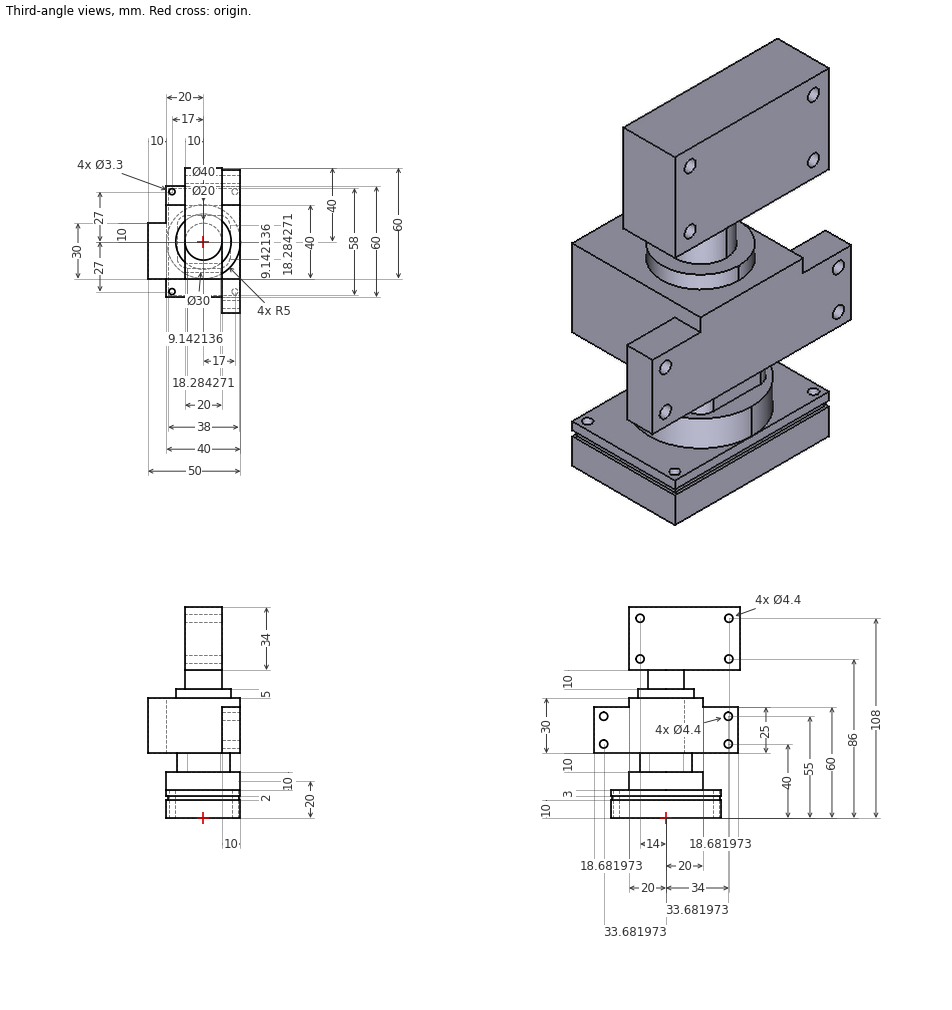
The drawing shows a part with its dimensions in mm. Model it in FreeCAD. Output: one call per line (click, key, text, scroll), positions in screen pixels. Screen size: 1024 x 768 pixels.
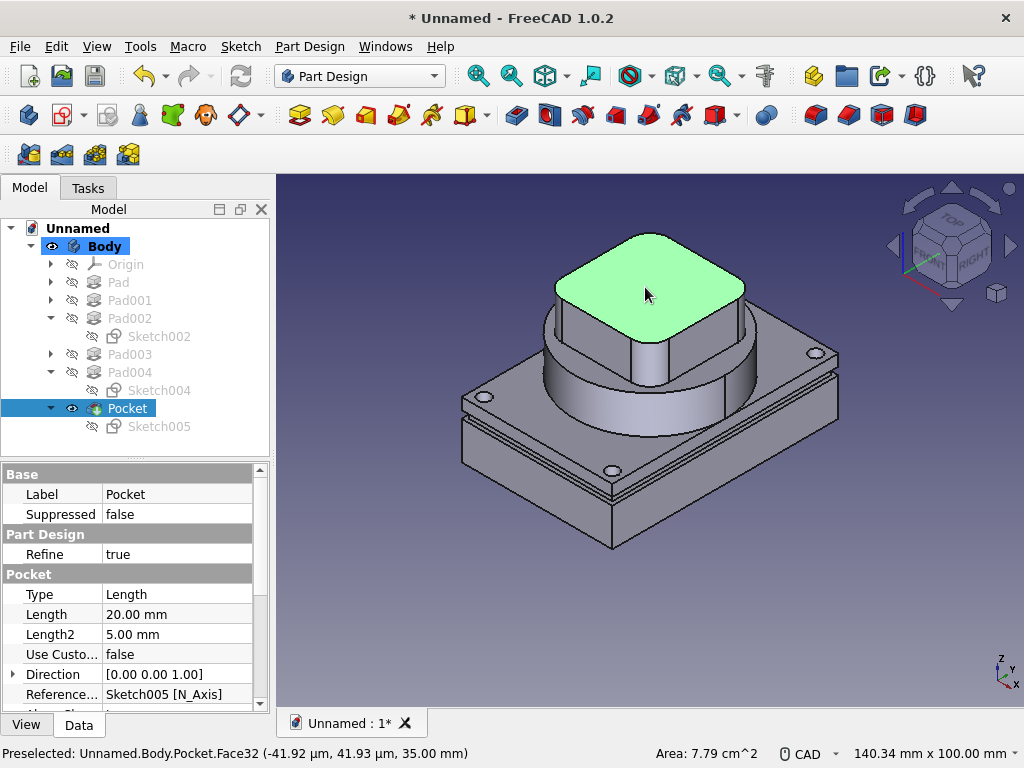
click(62, 116)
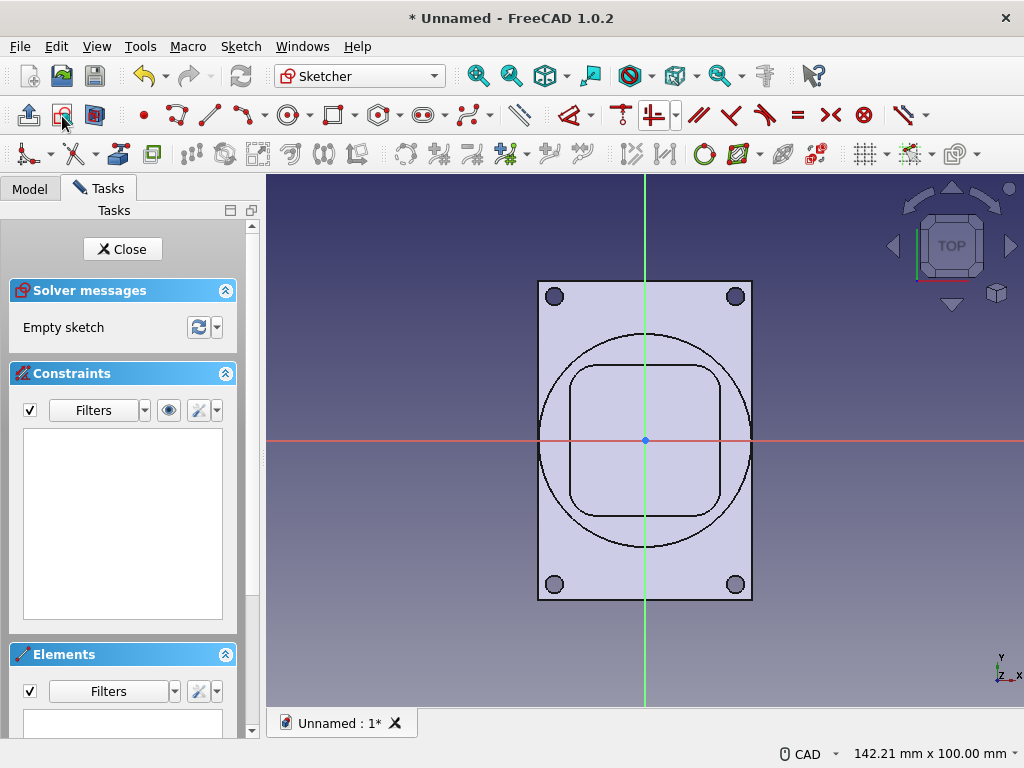
scroll(703, 440, up, 2)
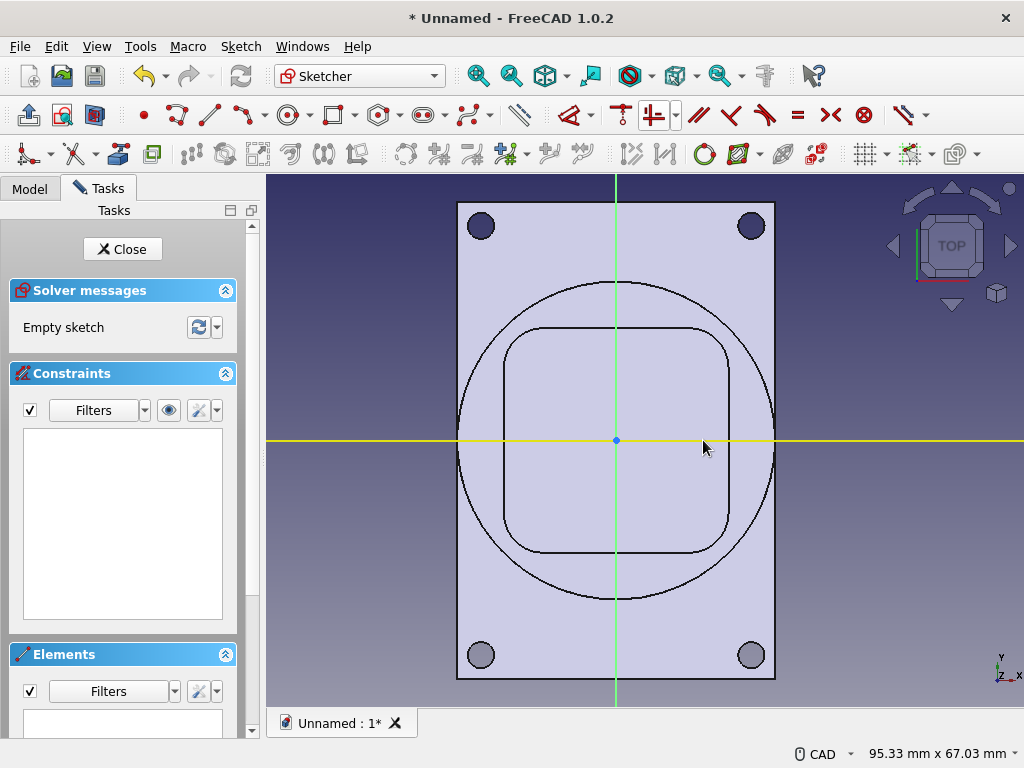
key(g)
key(m)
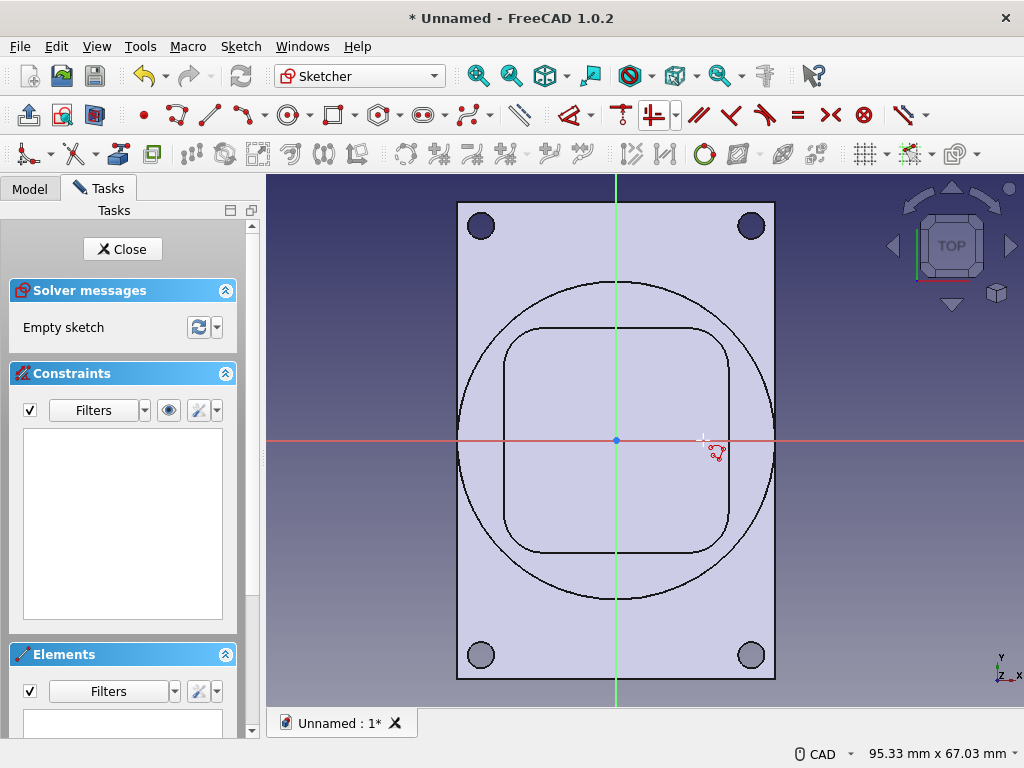
click(457, 361)
click(378, 361)
click(378, 600)
click(775, 600)
click(775, 281)
click(457, 281)
click(457, 362)
key(Escape)
key(Escape)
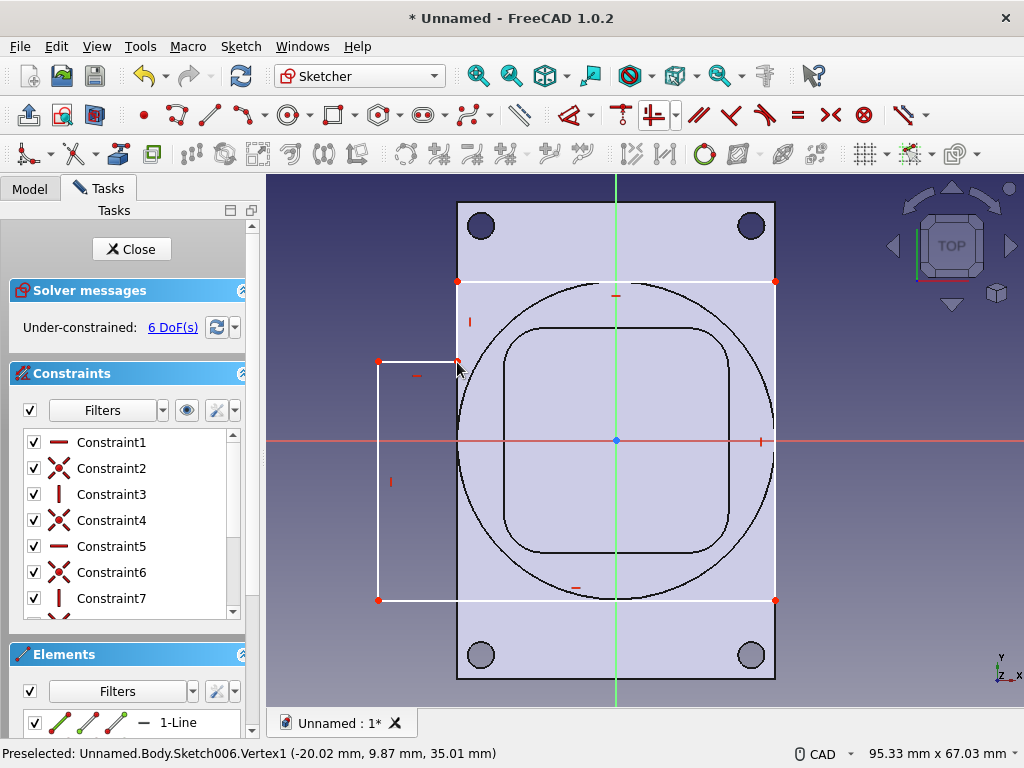
key(d)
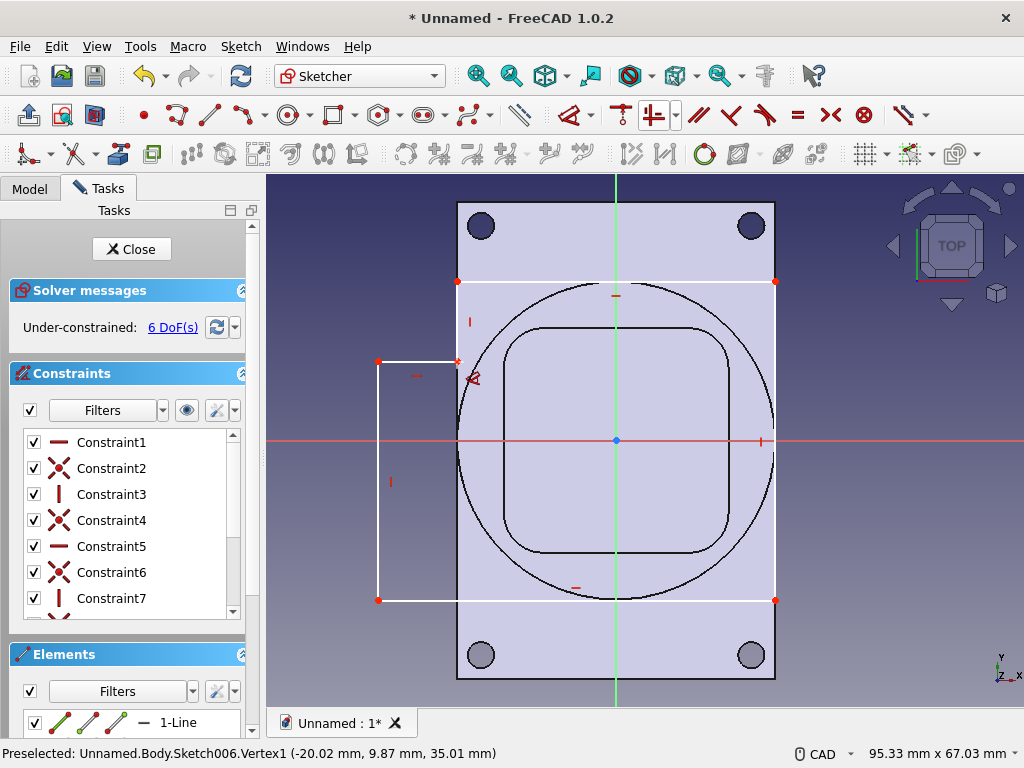
click(433, 362)
click(418, 328)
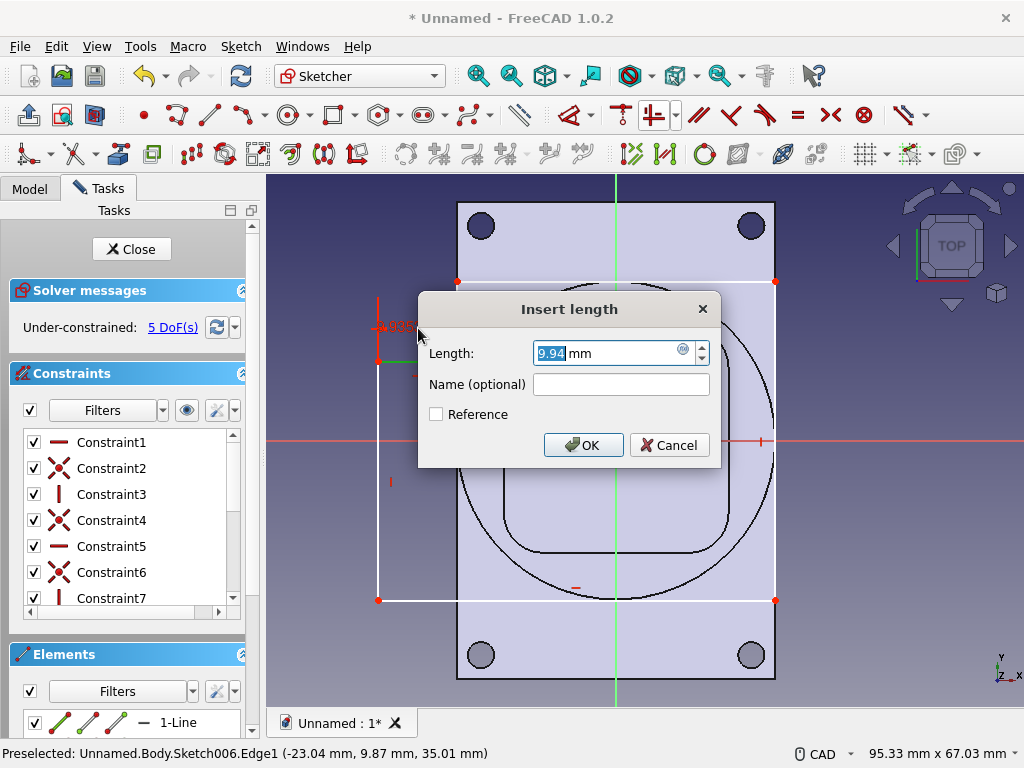
text(10)
key(Return)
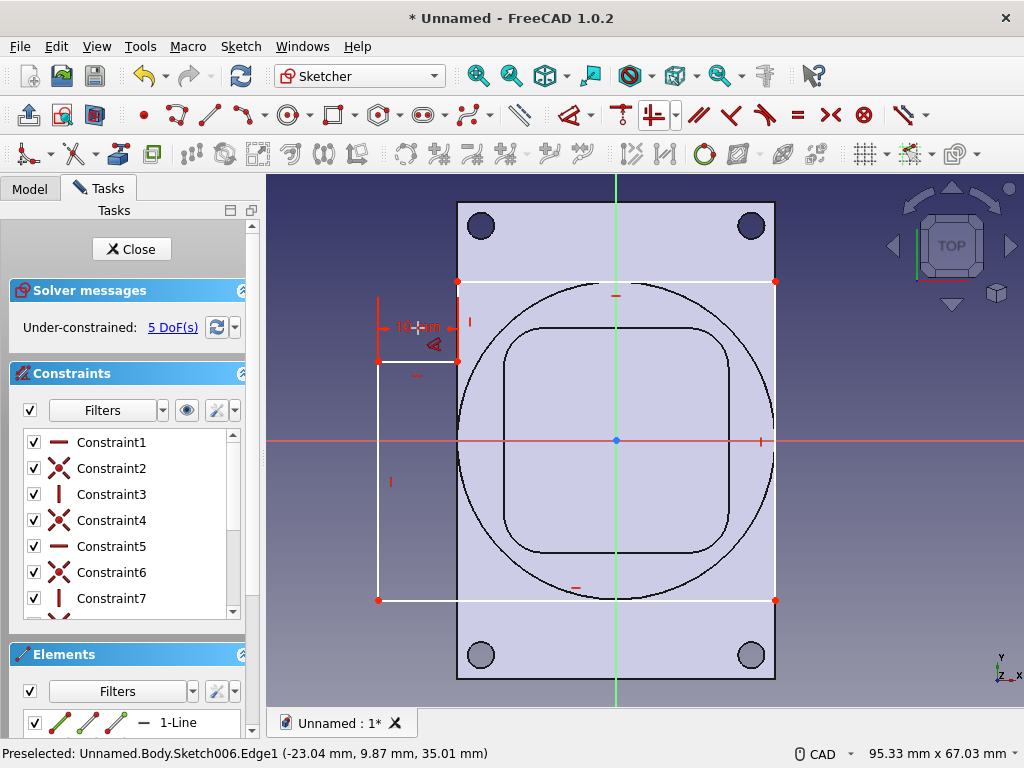
click(378, 529)
click(344, 481)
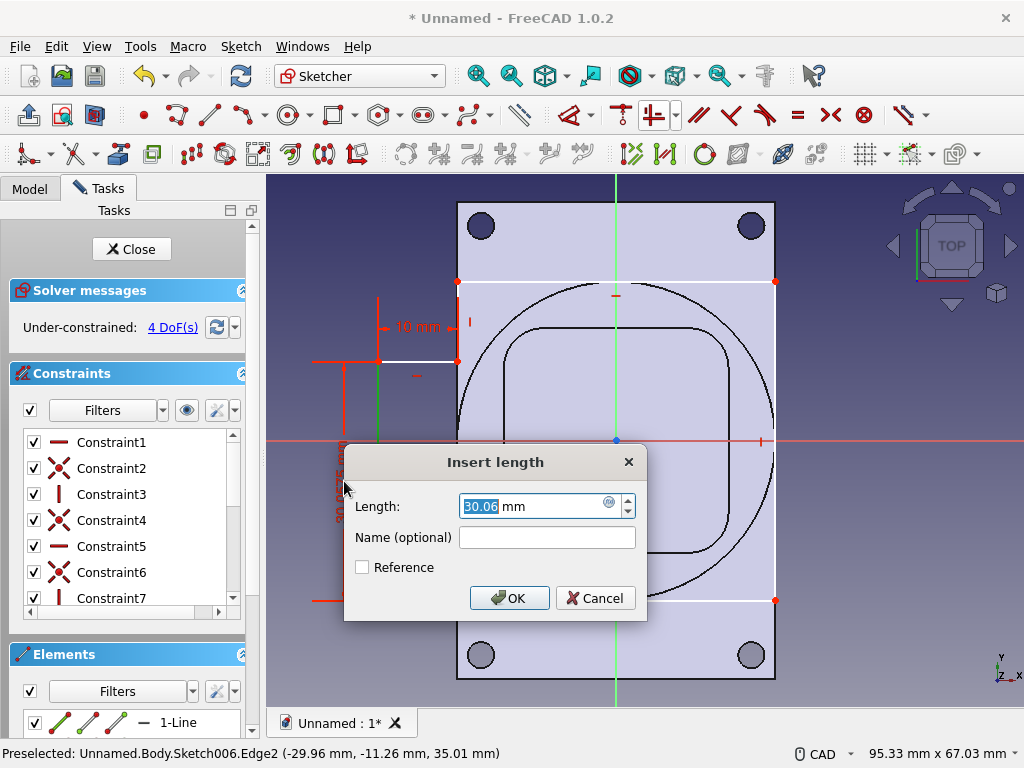
text(30)
key(Return)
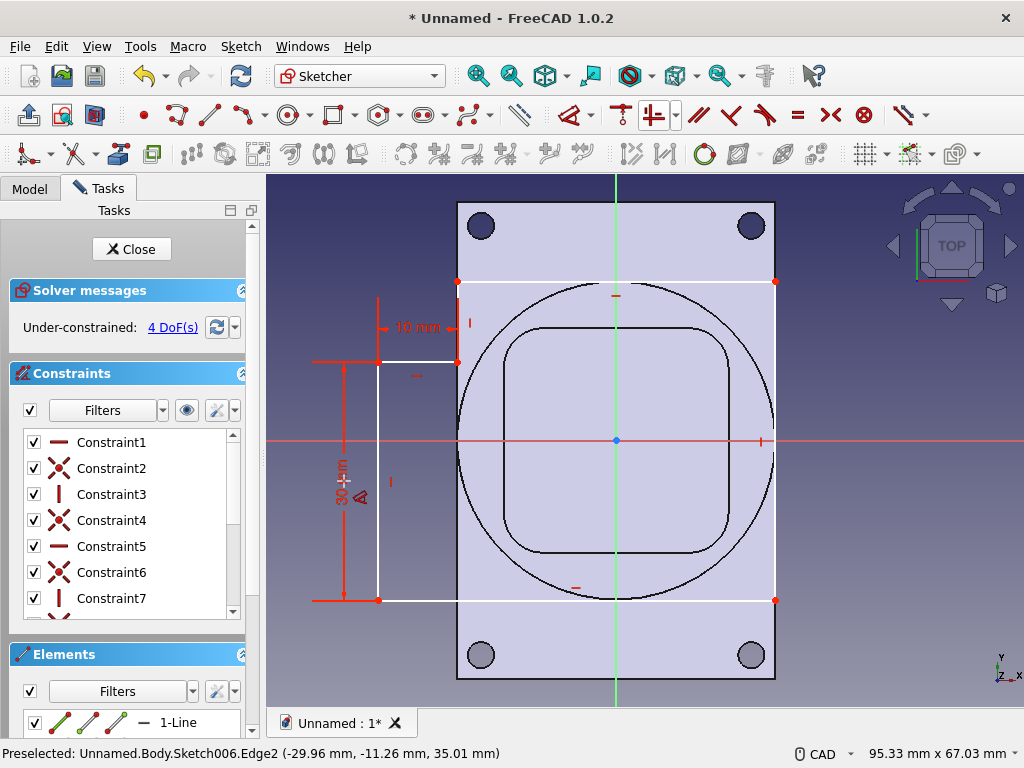
click(497, 601)
click(577, 635)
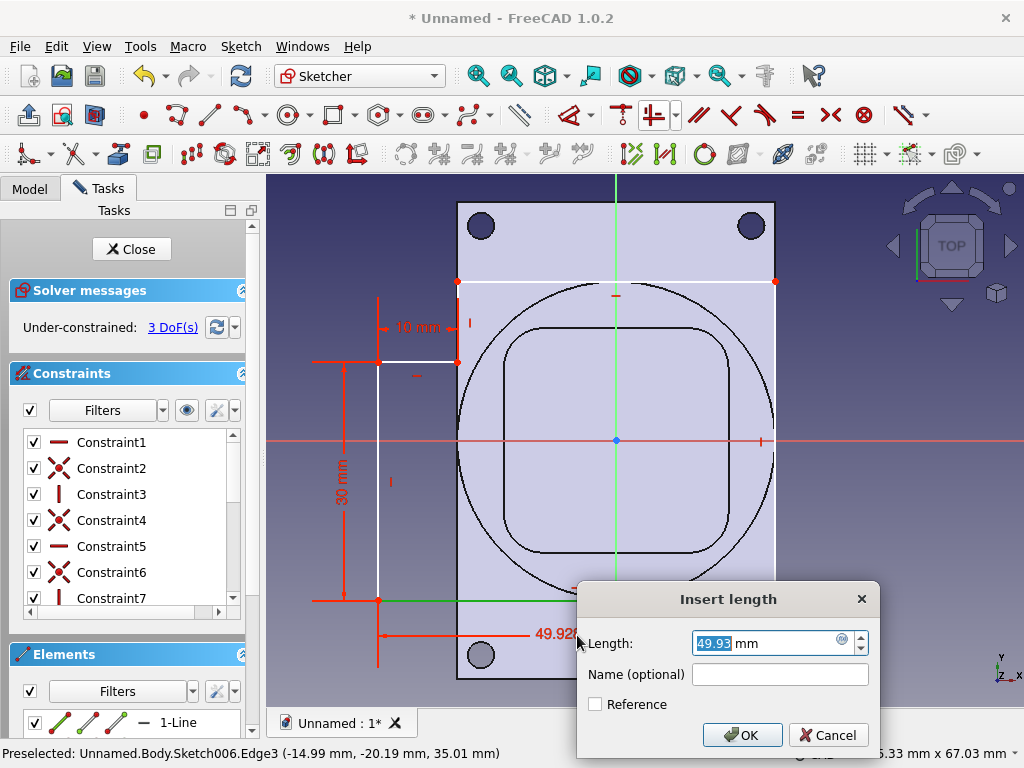
text(50)
key(Return)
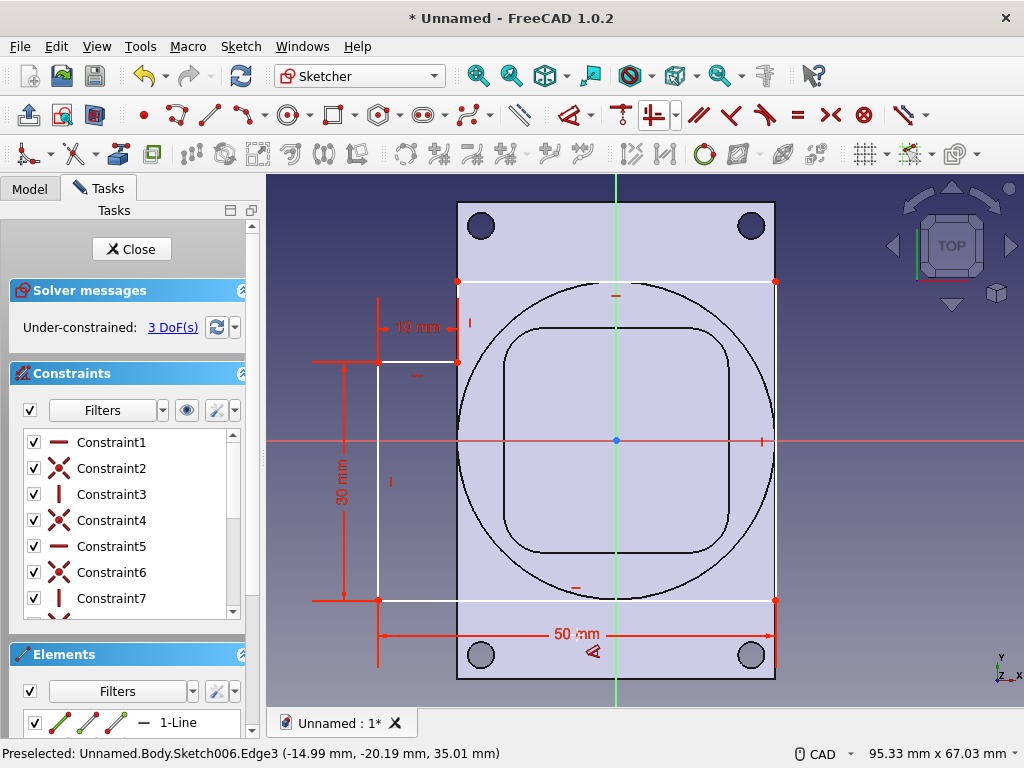
click(776, 505)
click(810, 368)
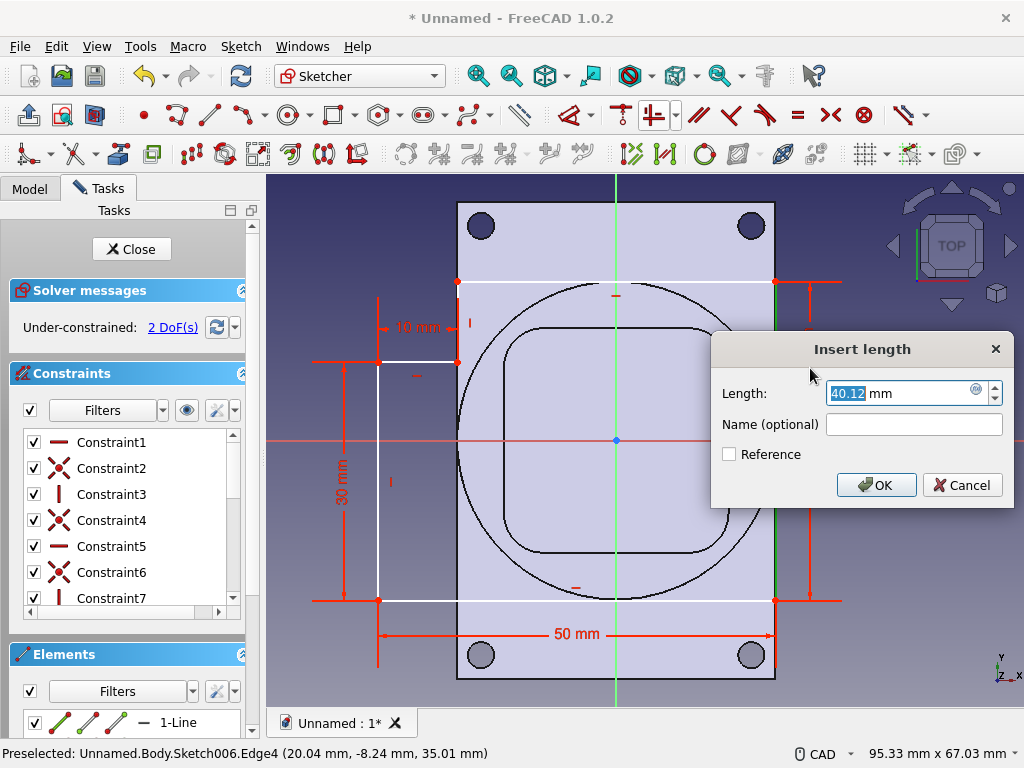
text(40)
key(Return)